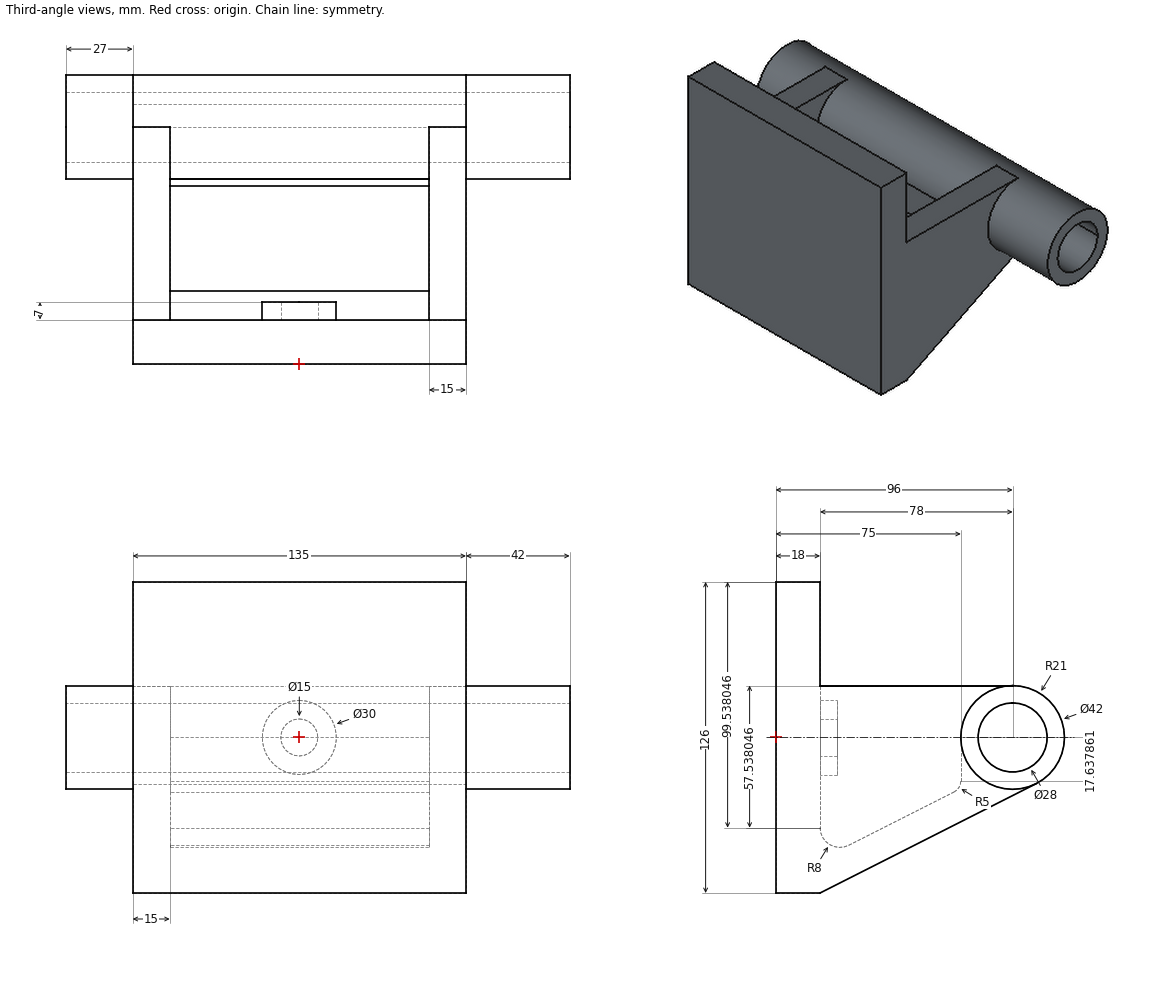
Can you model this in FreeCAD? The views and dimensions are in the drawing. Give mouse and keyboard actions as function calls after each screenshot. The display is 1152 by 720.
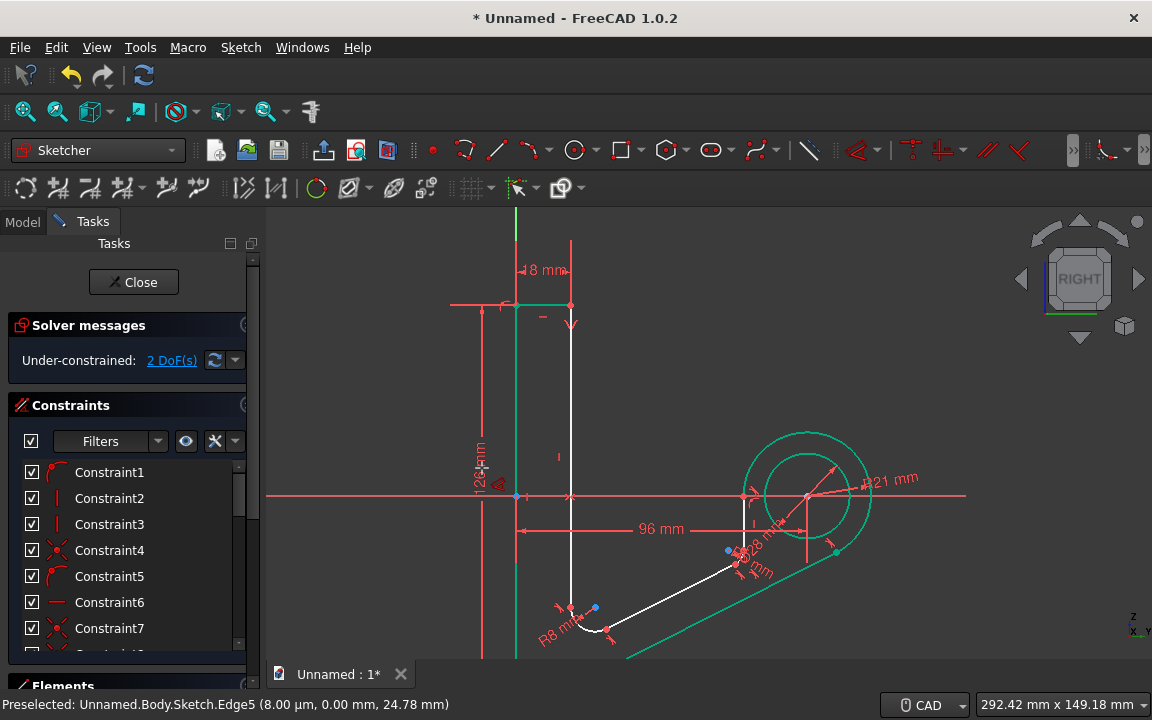
click(744, 512)
click(802, 511)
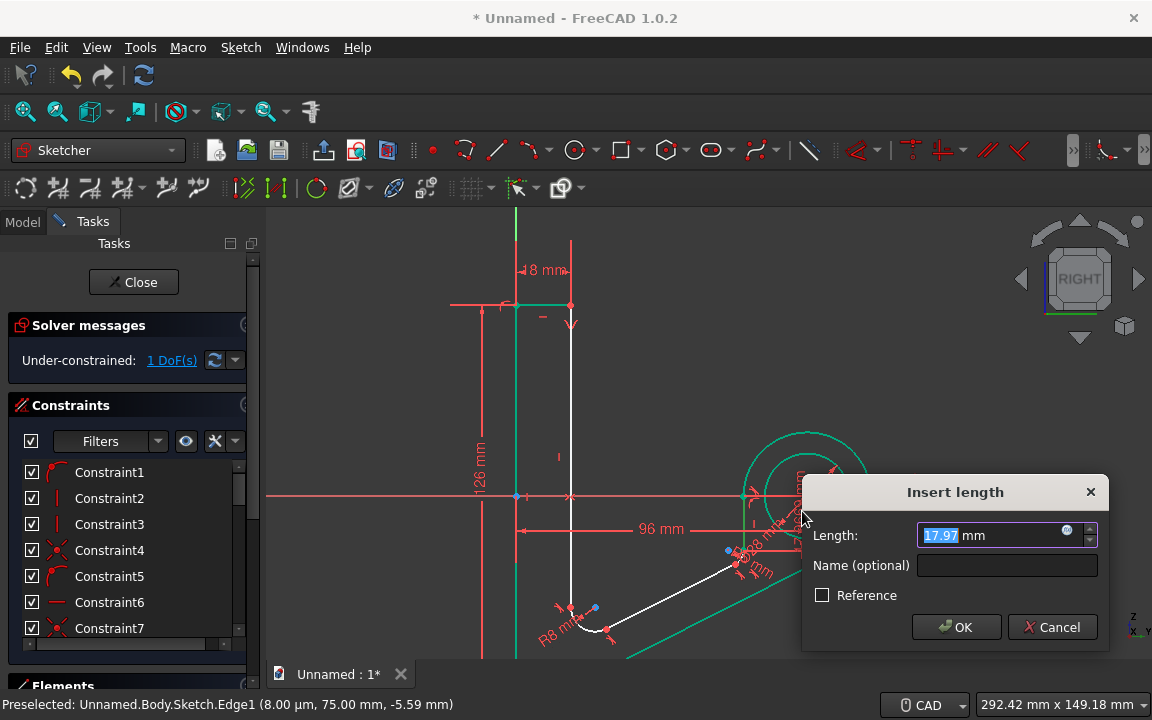
text(17.637861)
key(Return)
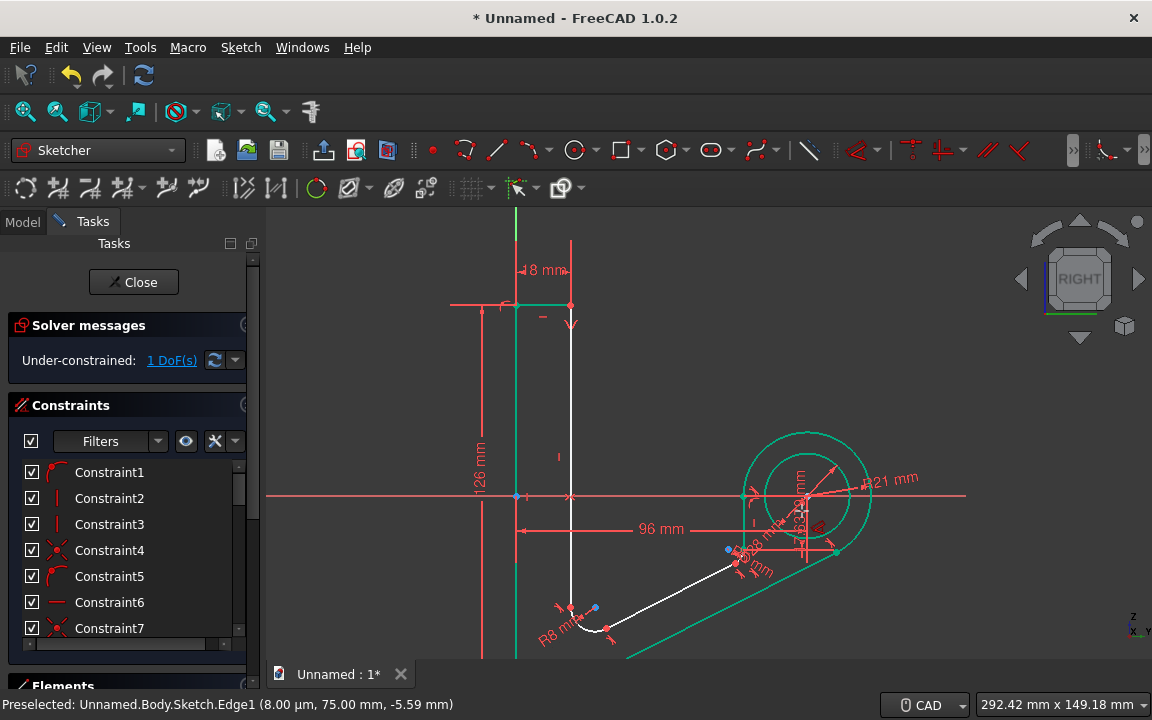
click(571, 517)
click(537, 387)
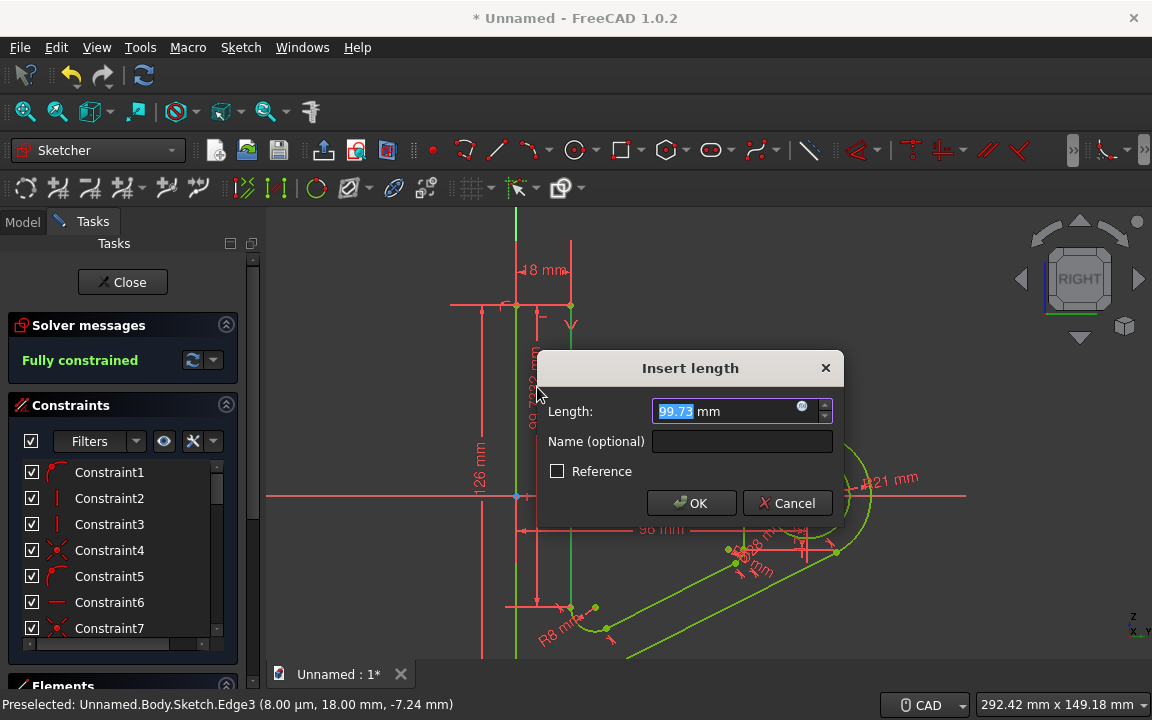
text(99.538046)
key(Return)
key(Escape)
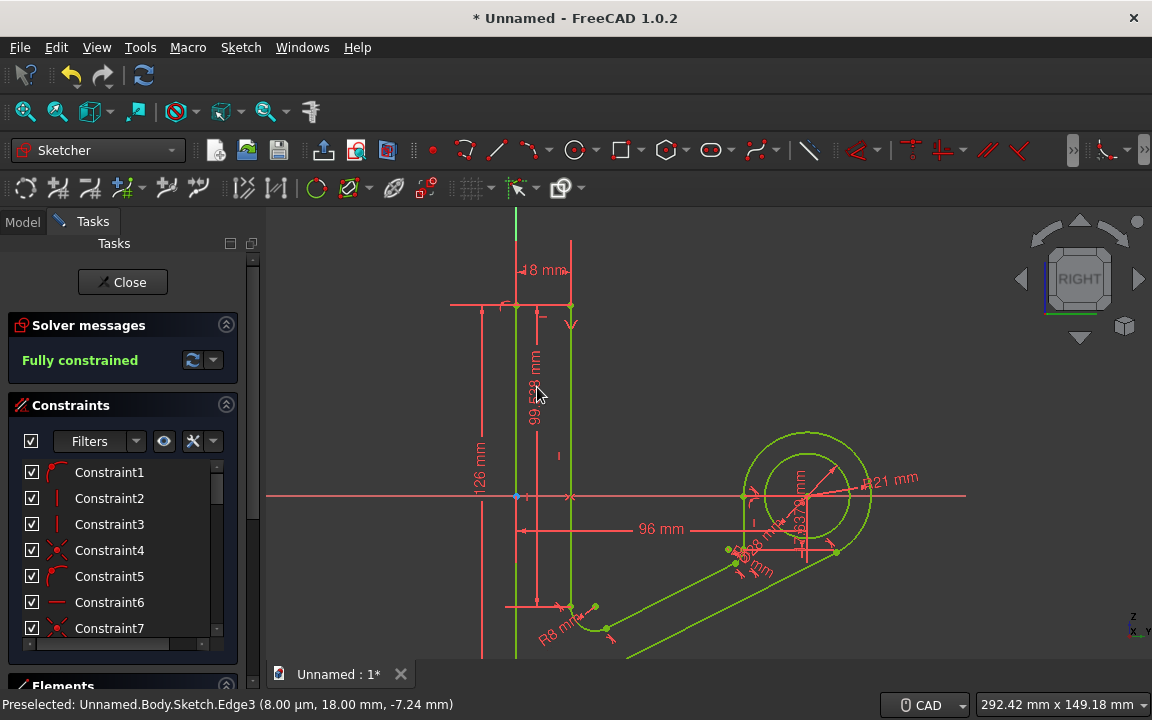
click(123, 282)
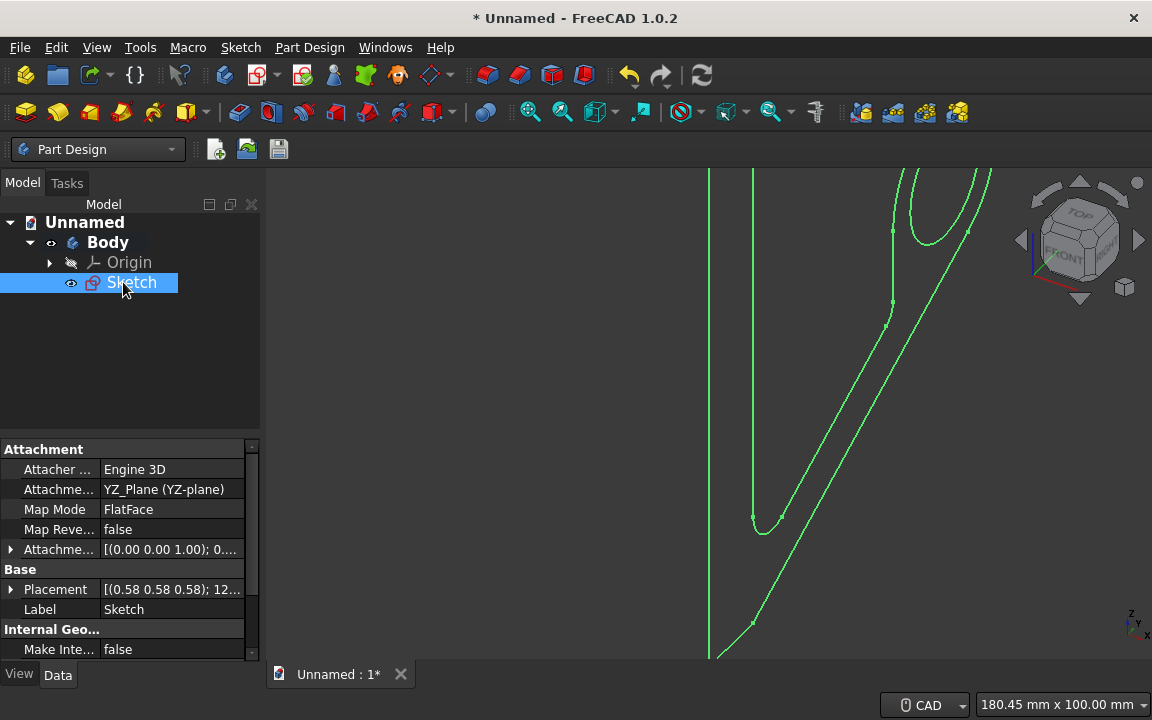
click(26, 112)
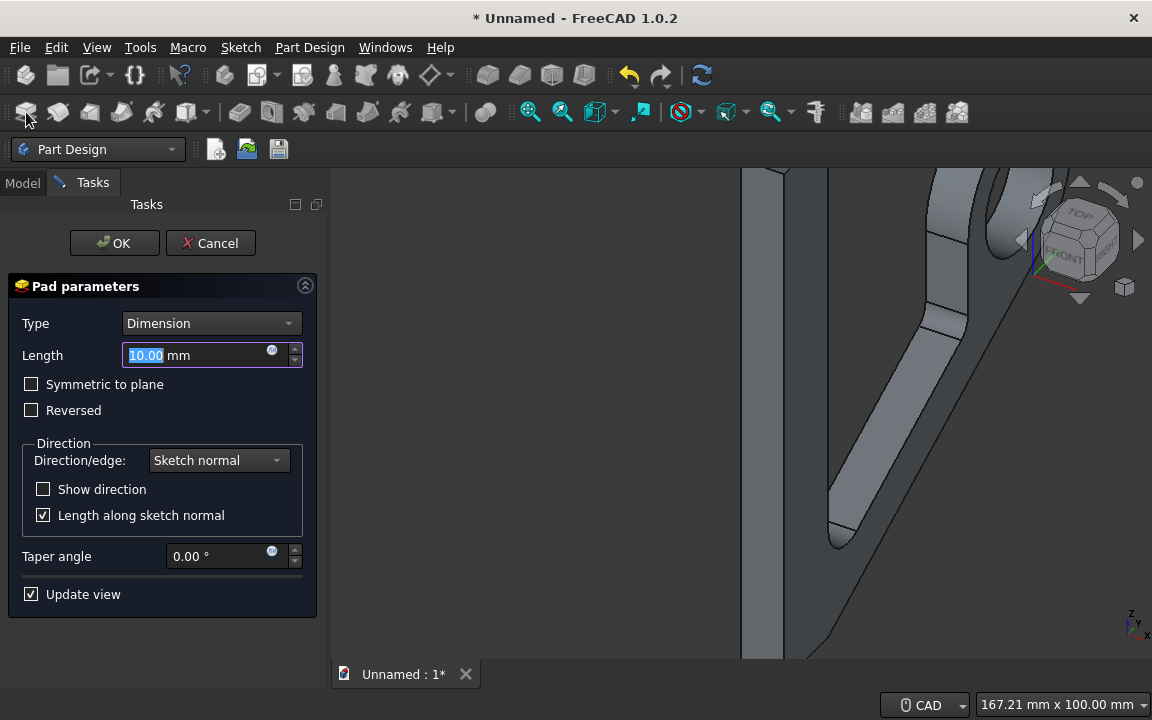
text(135)
key(Tab)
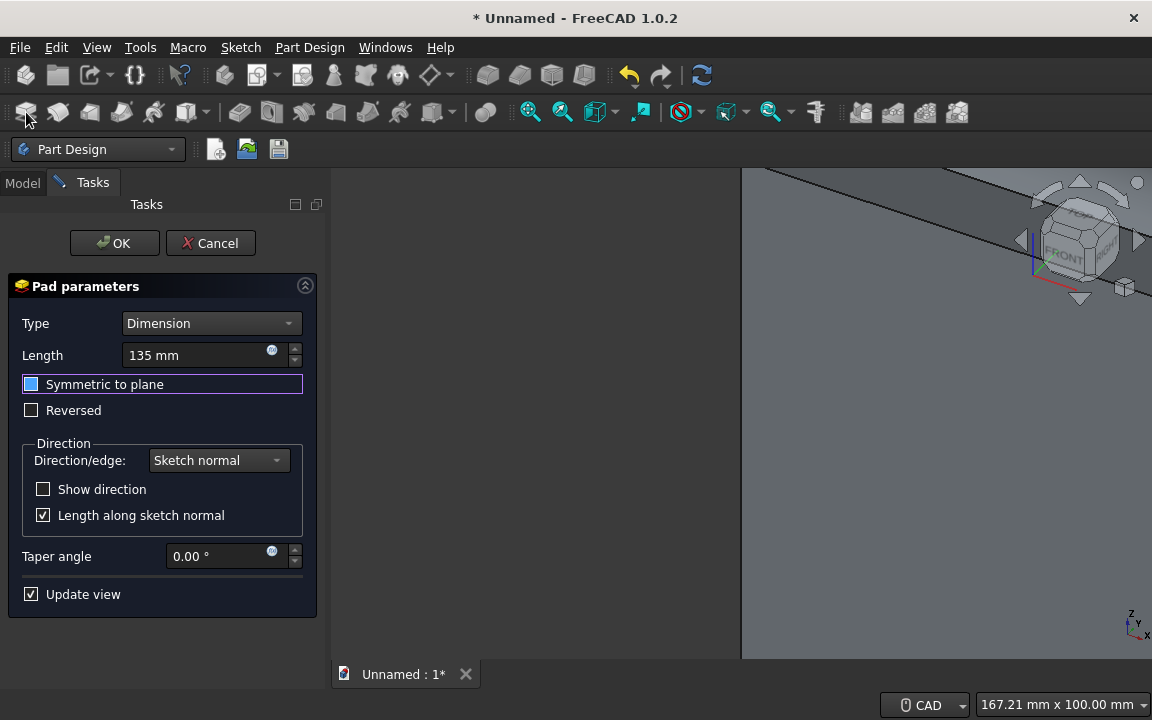
click(30, 384)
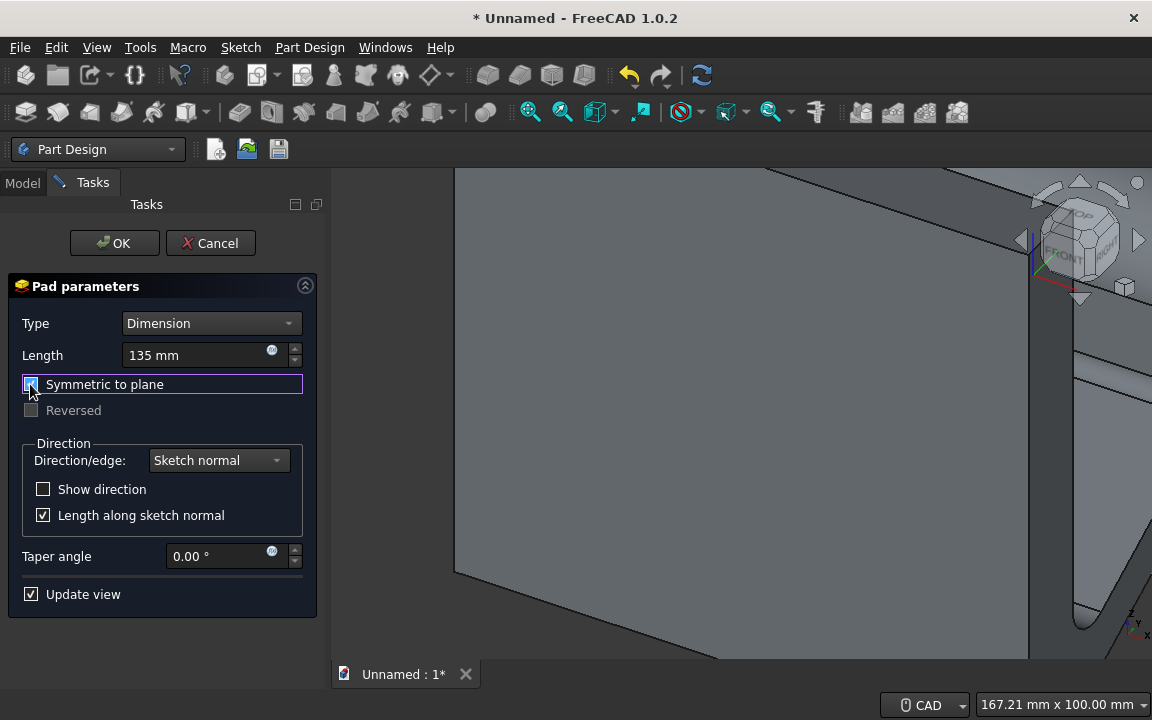
click(115, 243)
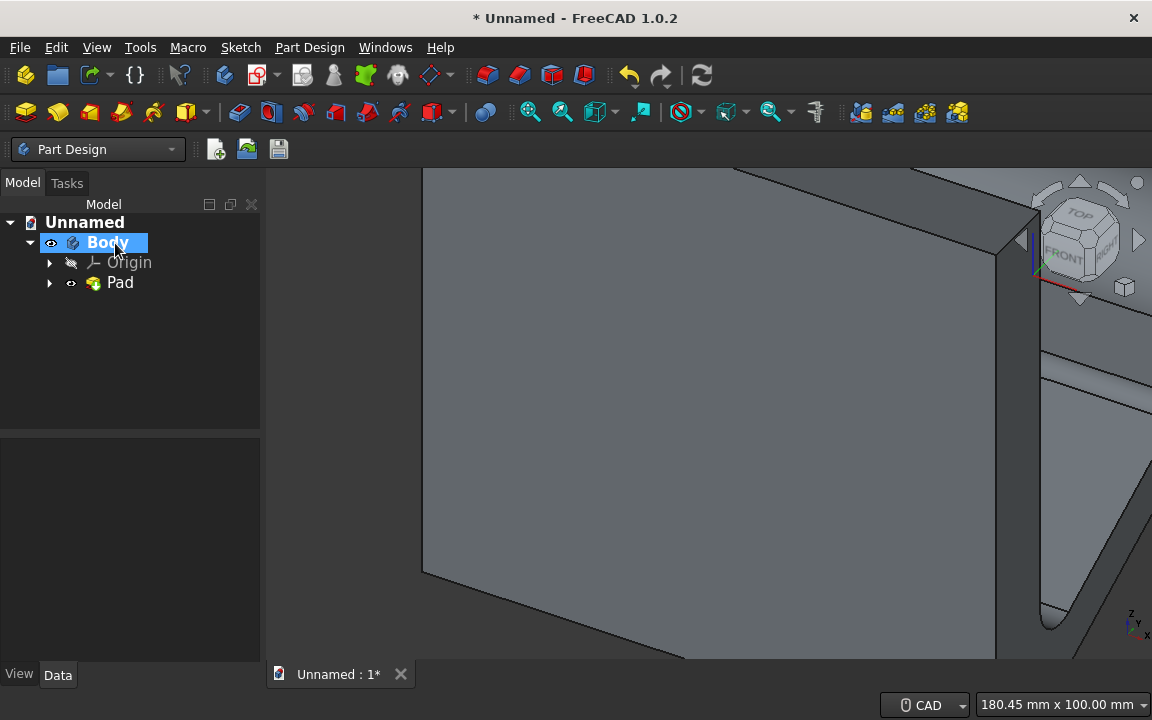
click(532, 112)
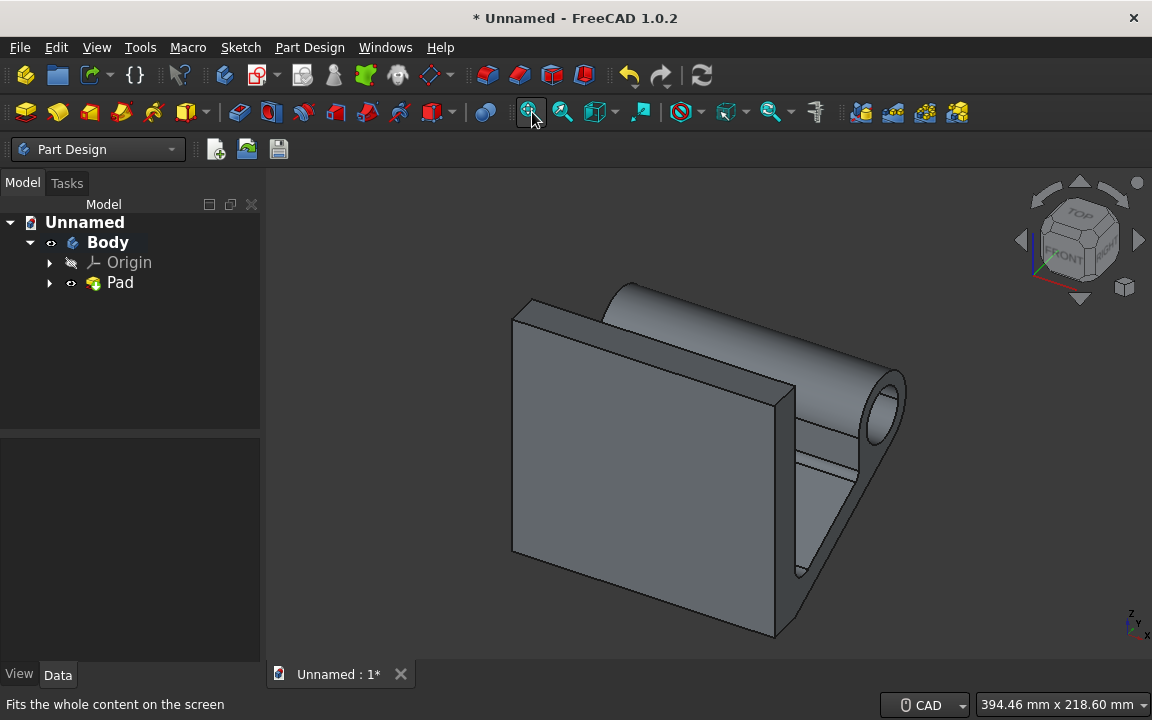
key(6)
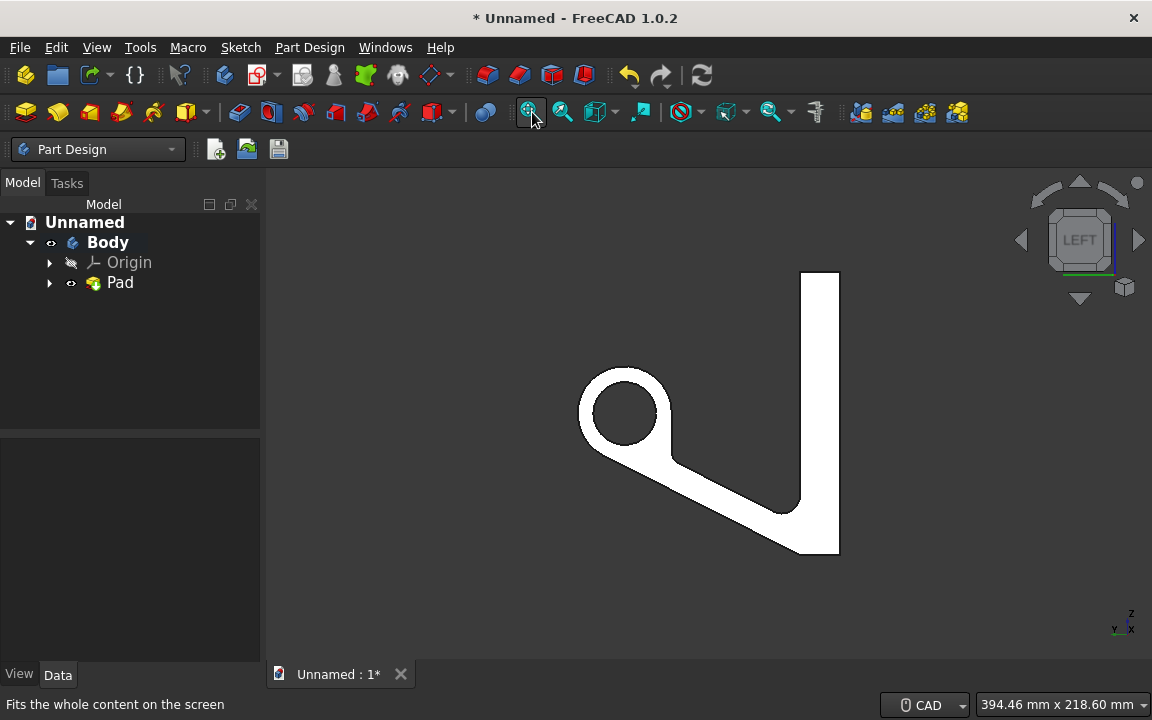
click(822, 493)